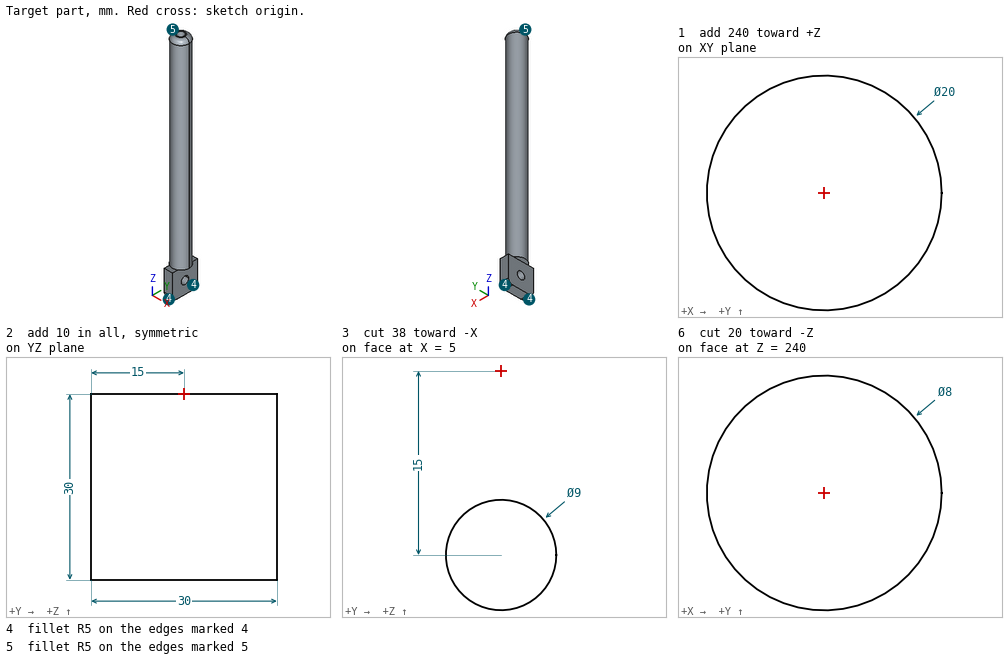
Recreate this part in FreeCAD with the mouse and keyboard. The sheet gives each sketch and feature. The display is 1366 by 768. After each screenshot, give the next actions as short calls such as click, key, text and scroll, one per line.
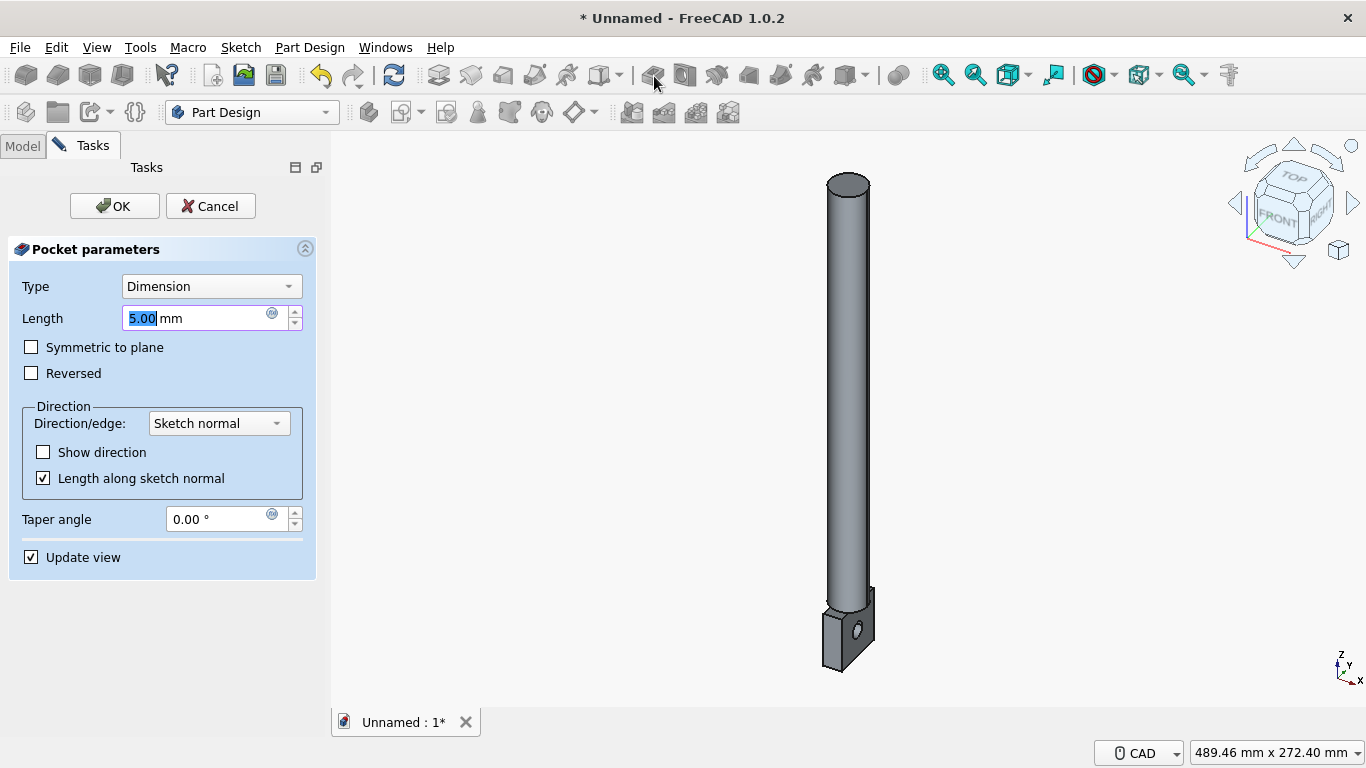
text(38)
key(Tab)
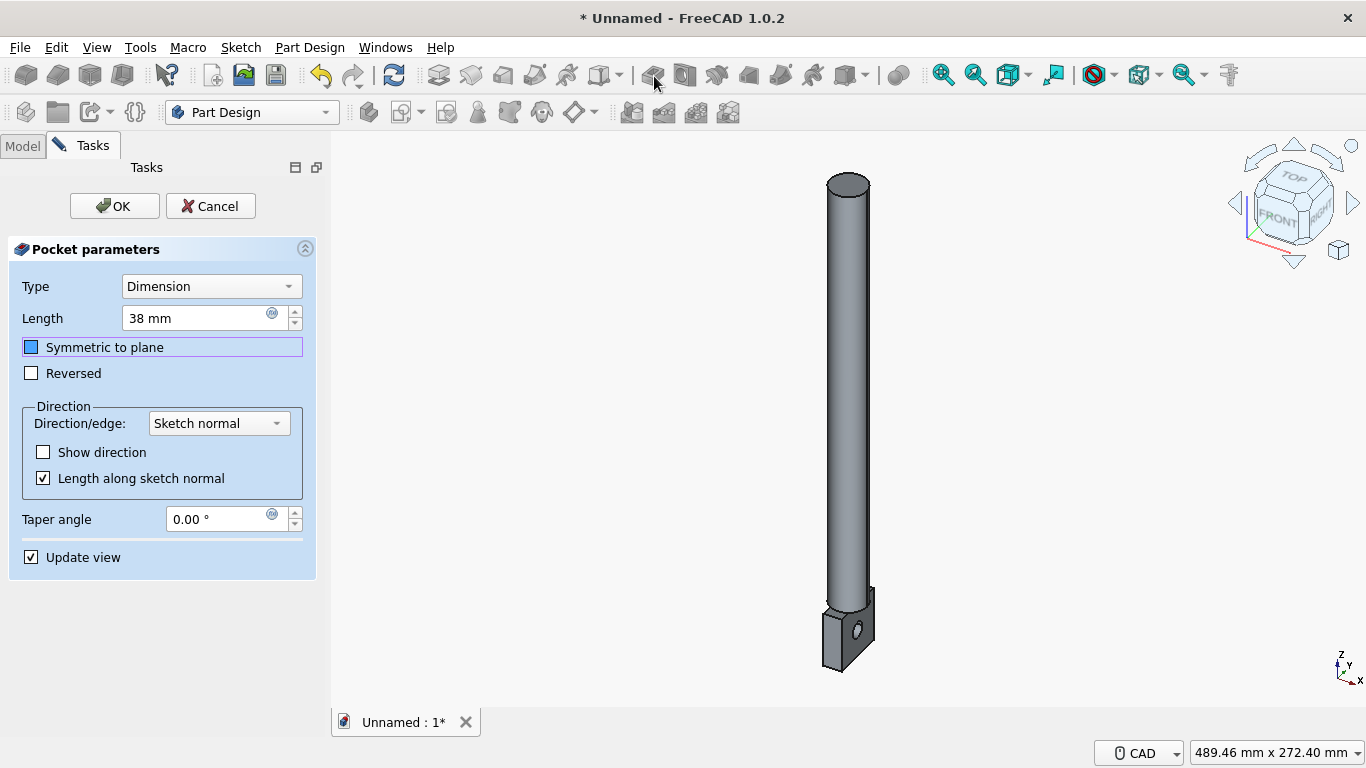
click(115, 206)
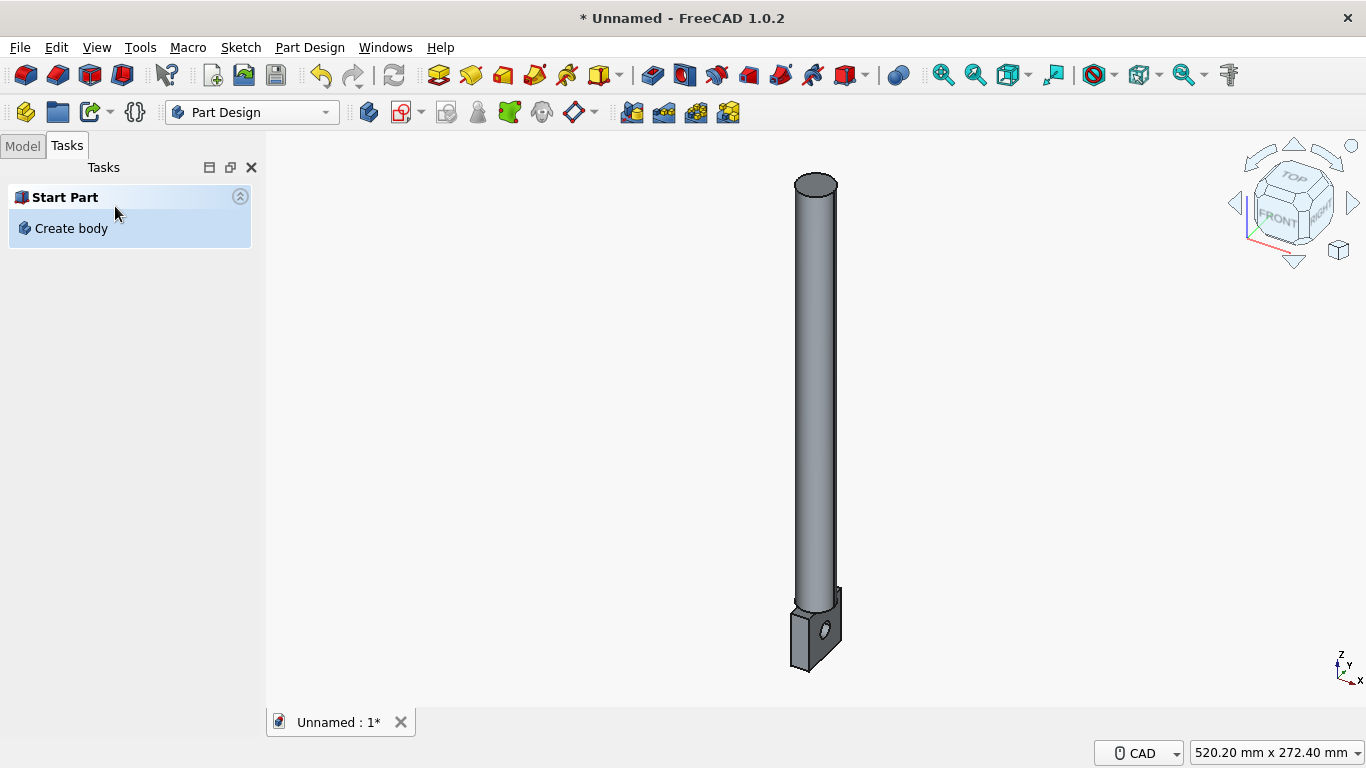
scroll(800, 668, up, 4)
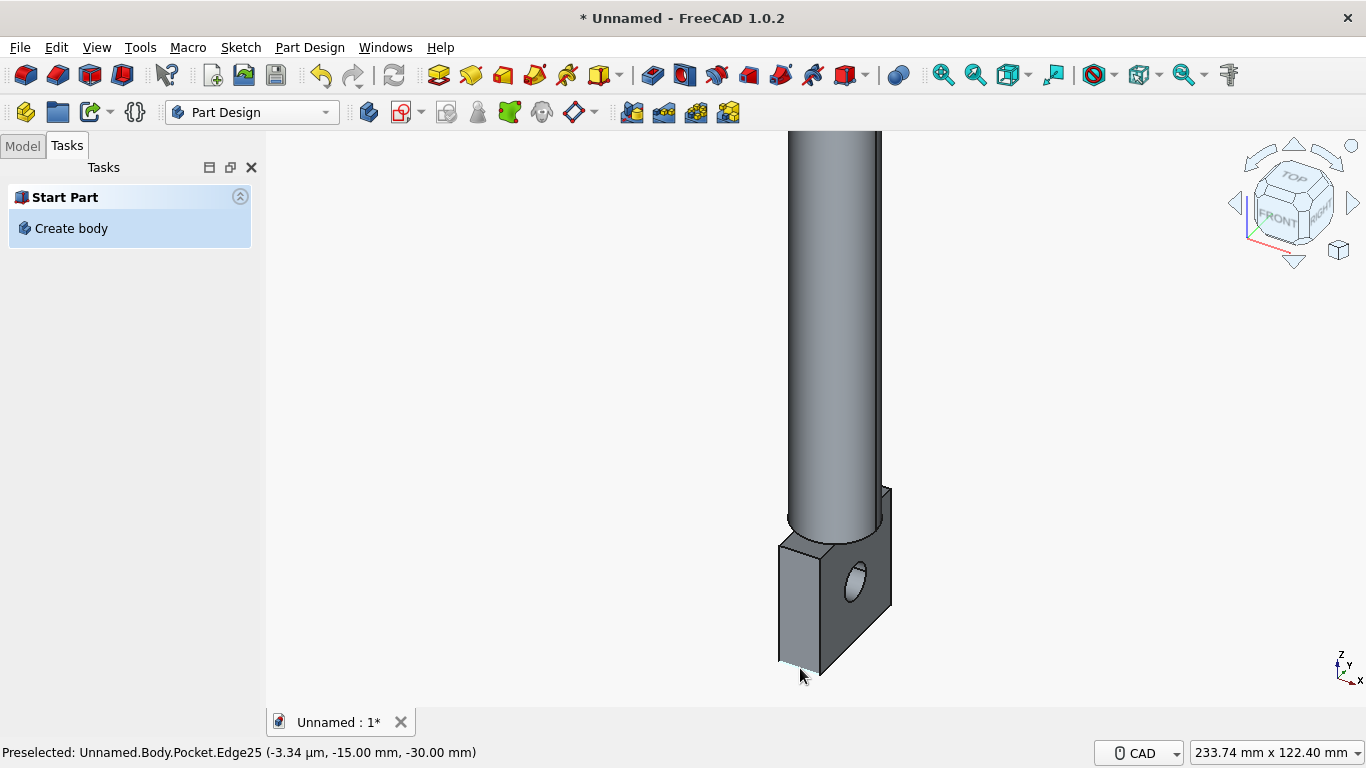
click(944, 76)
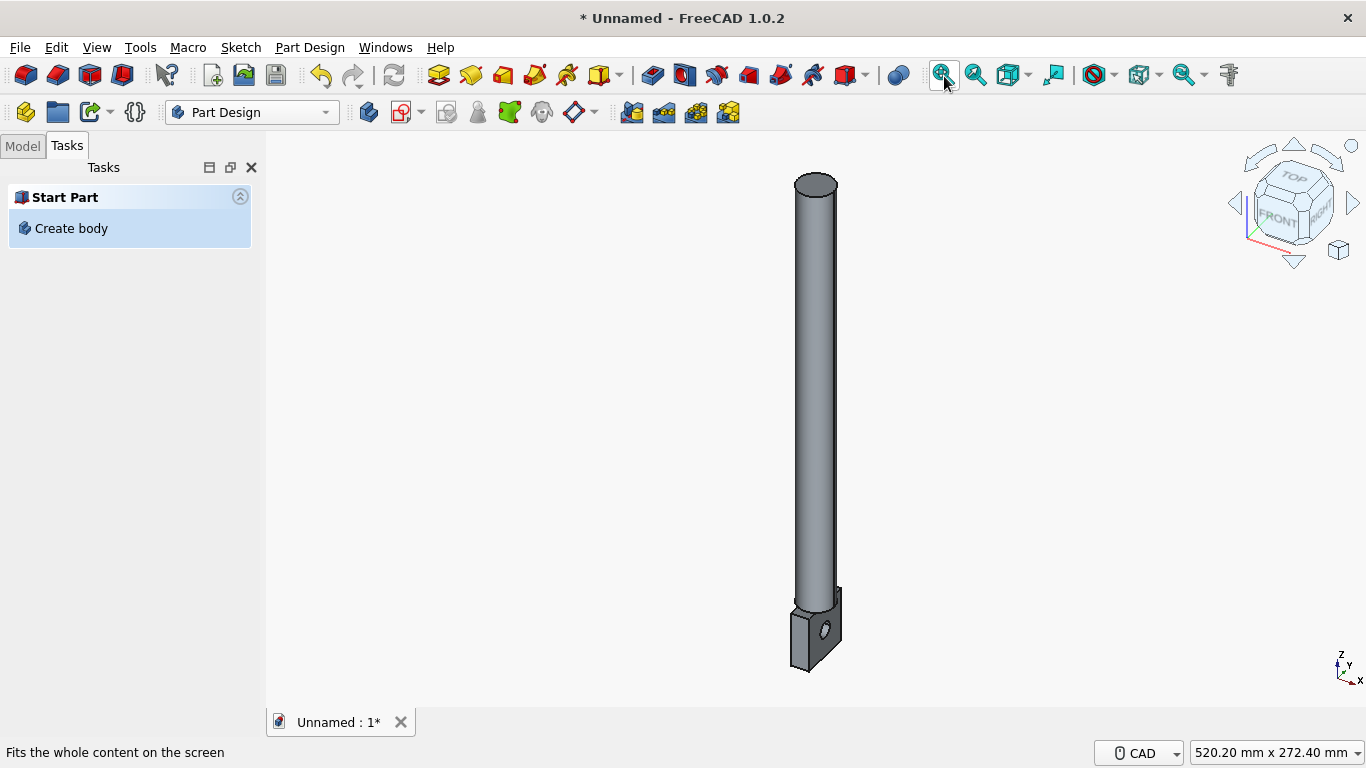
key(0)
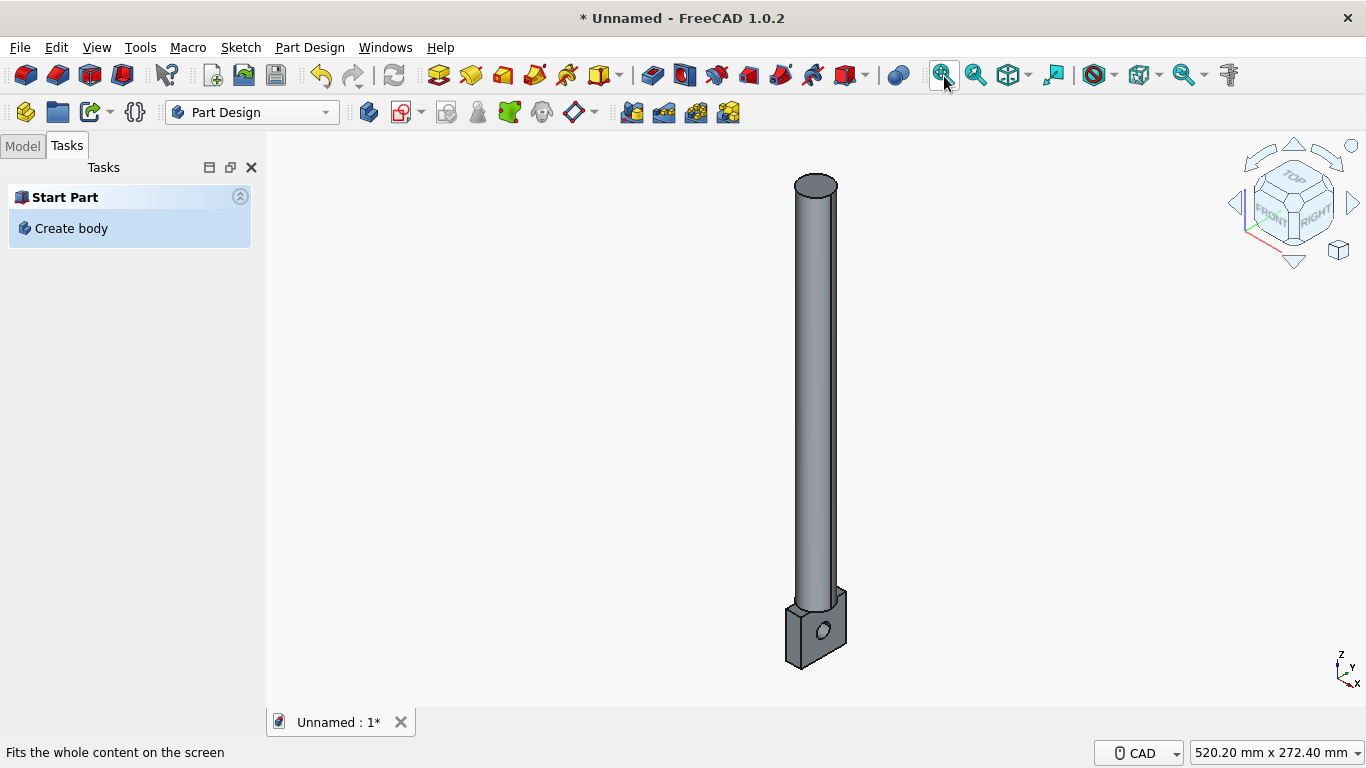
scroll(794, 664, up, 4)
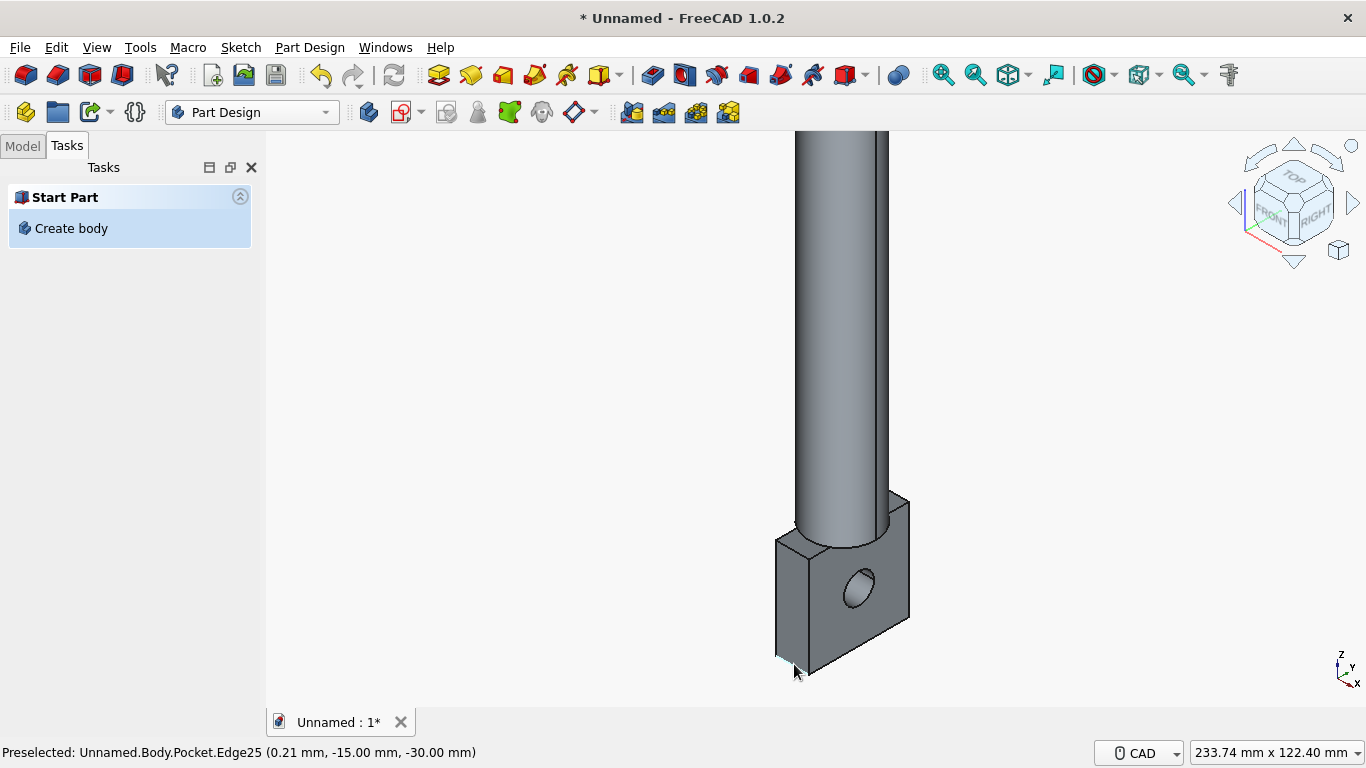
key(v)
key(f)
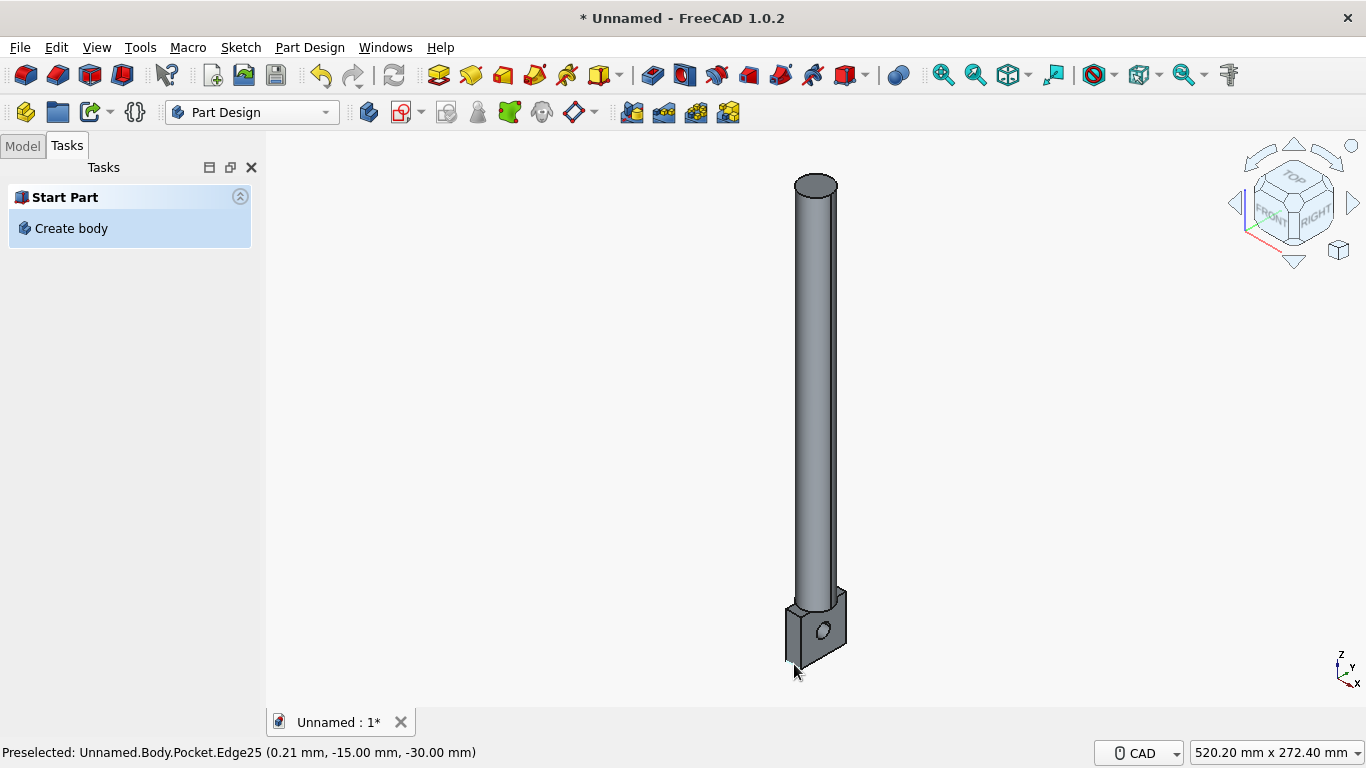
key(2)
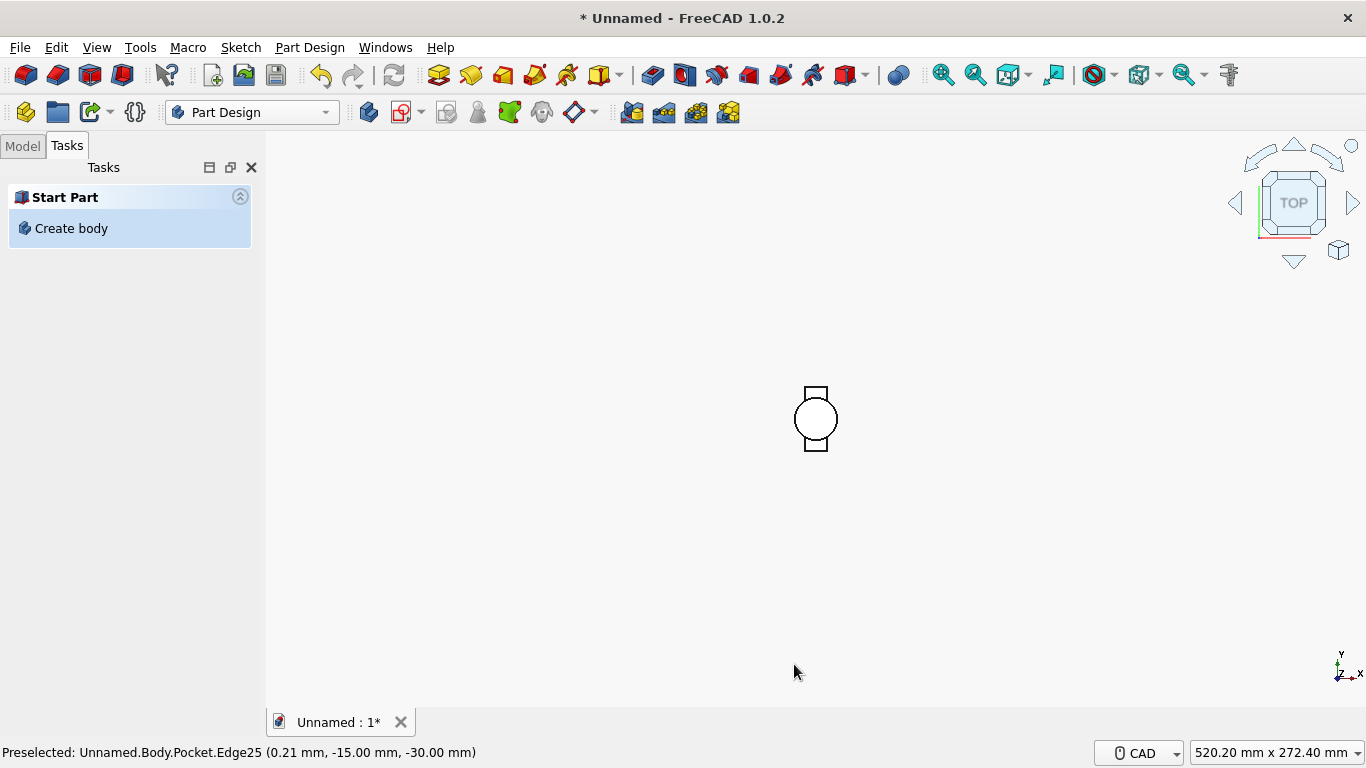
key(v)
key(f)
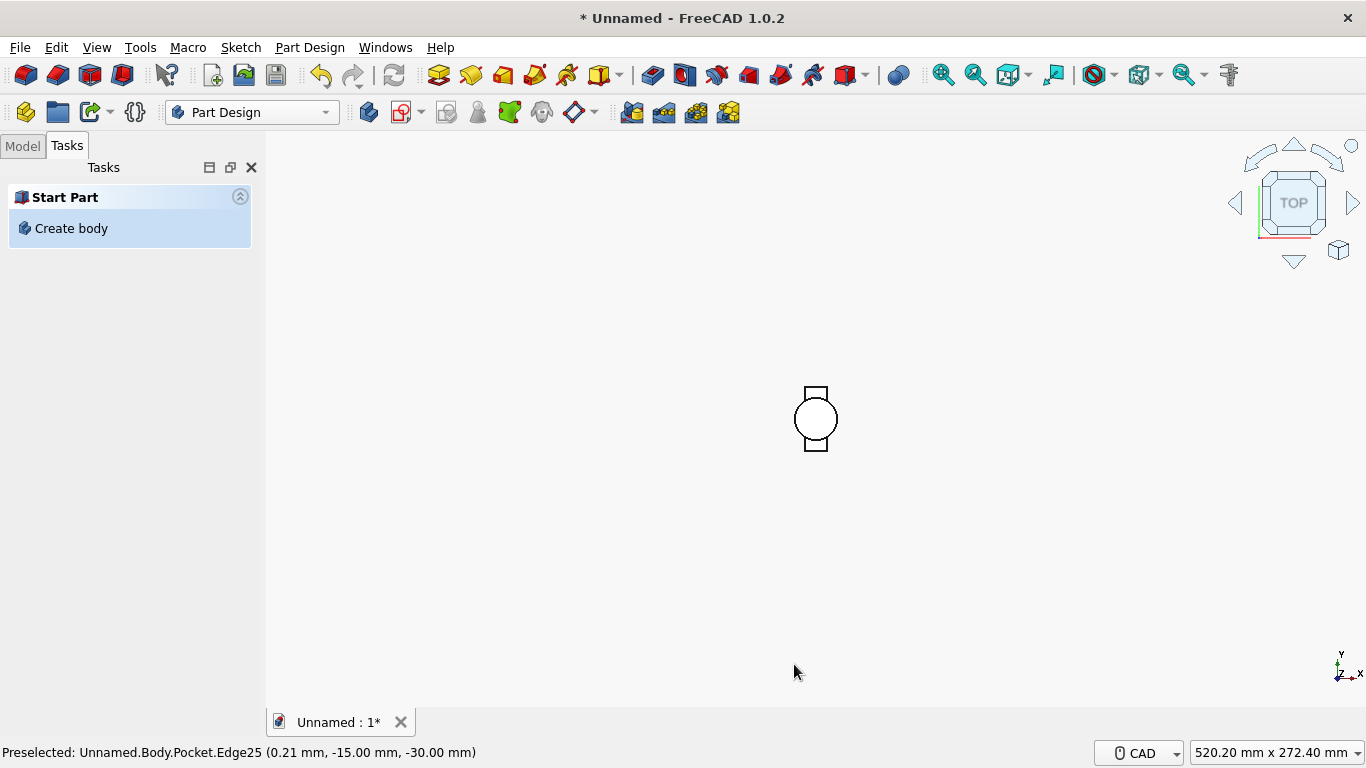
scroll(816, 450, up, 4)